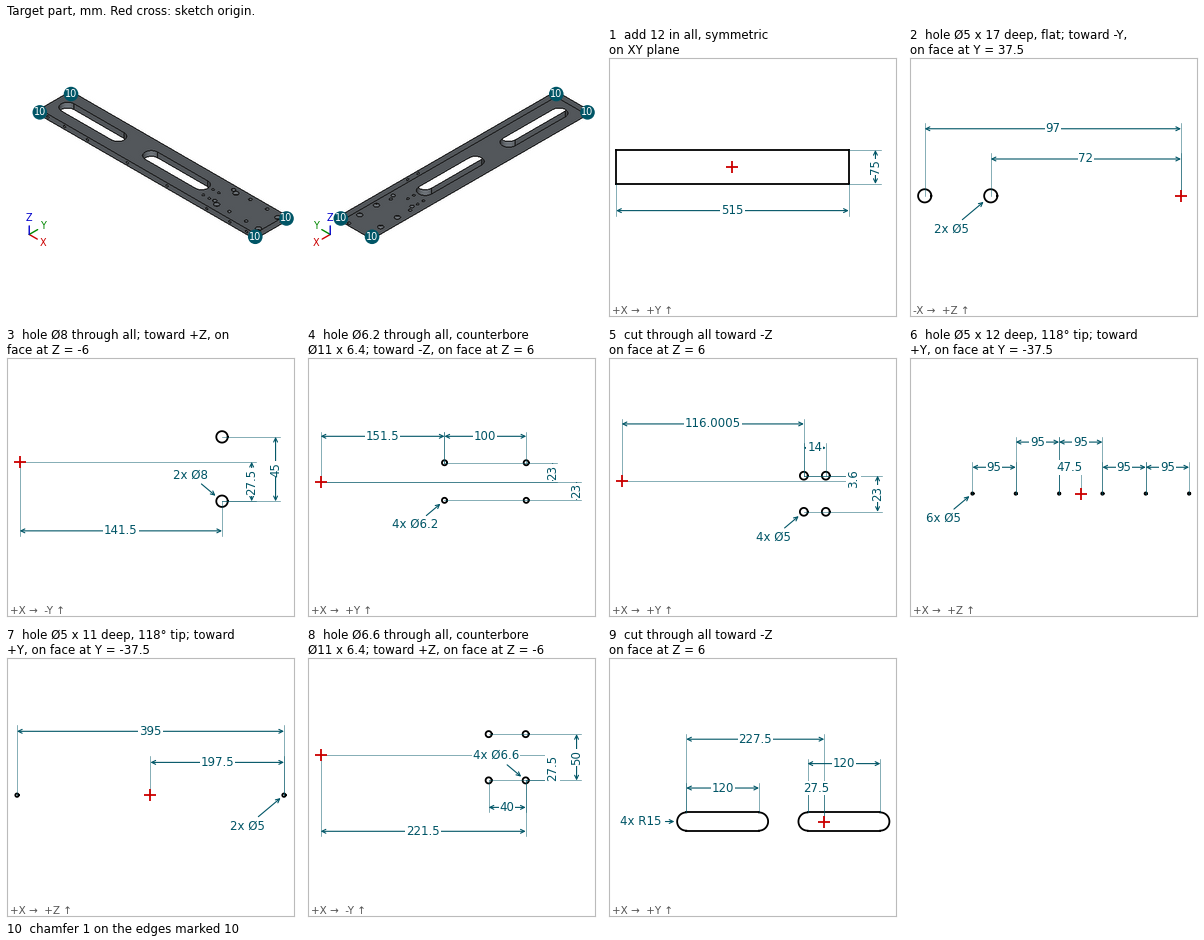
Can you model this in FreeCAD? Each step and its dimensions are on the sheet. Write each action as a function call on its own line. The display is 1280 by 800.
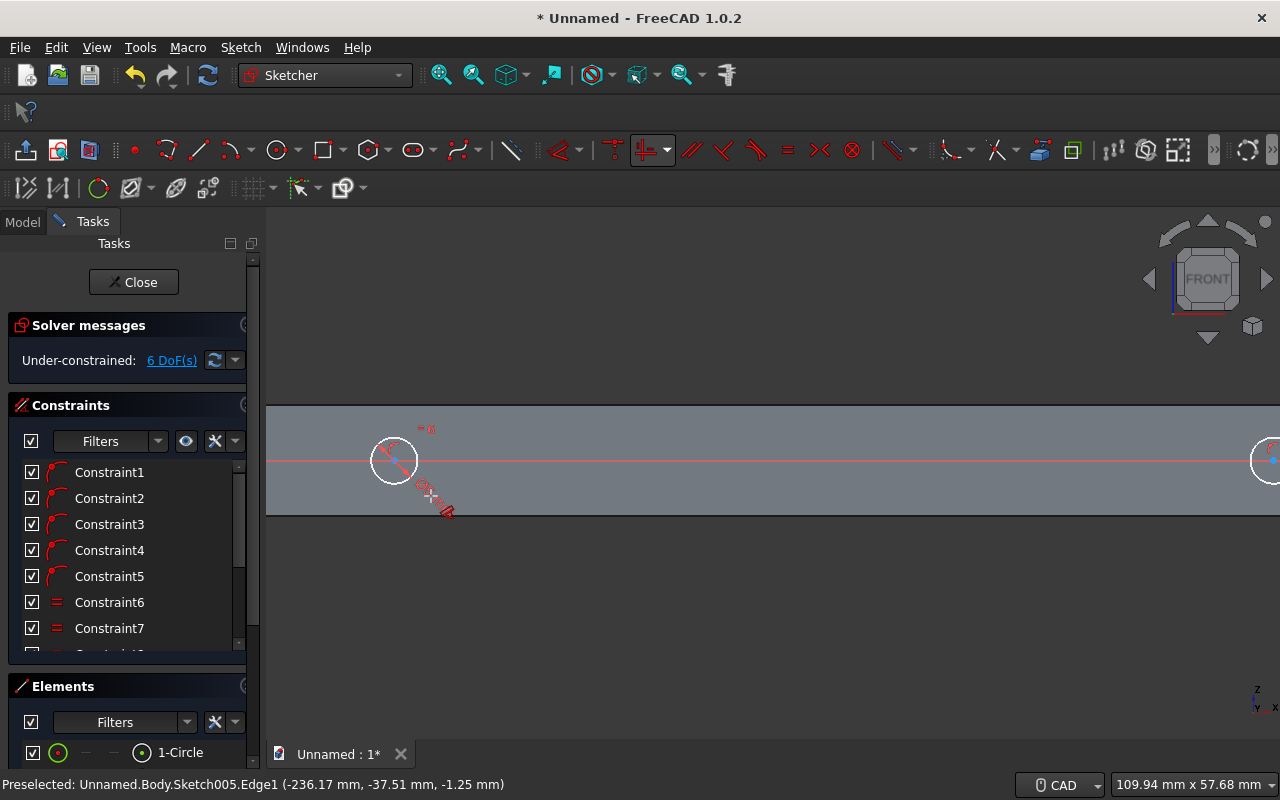
scroll(410, 475, down, 10)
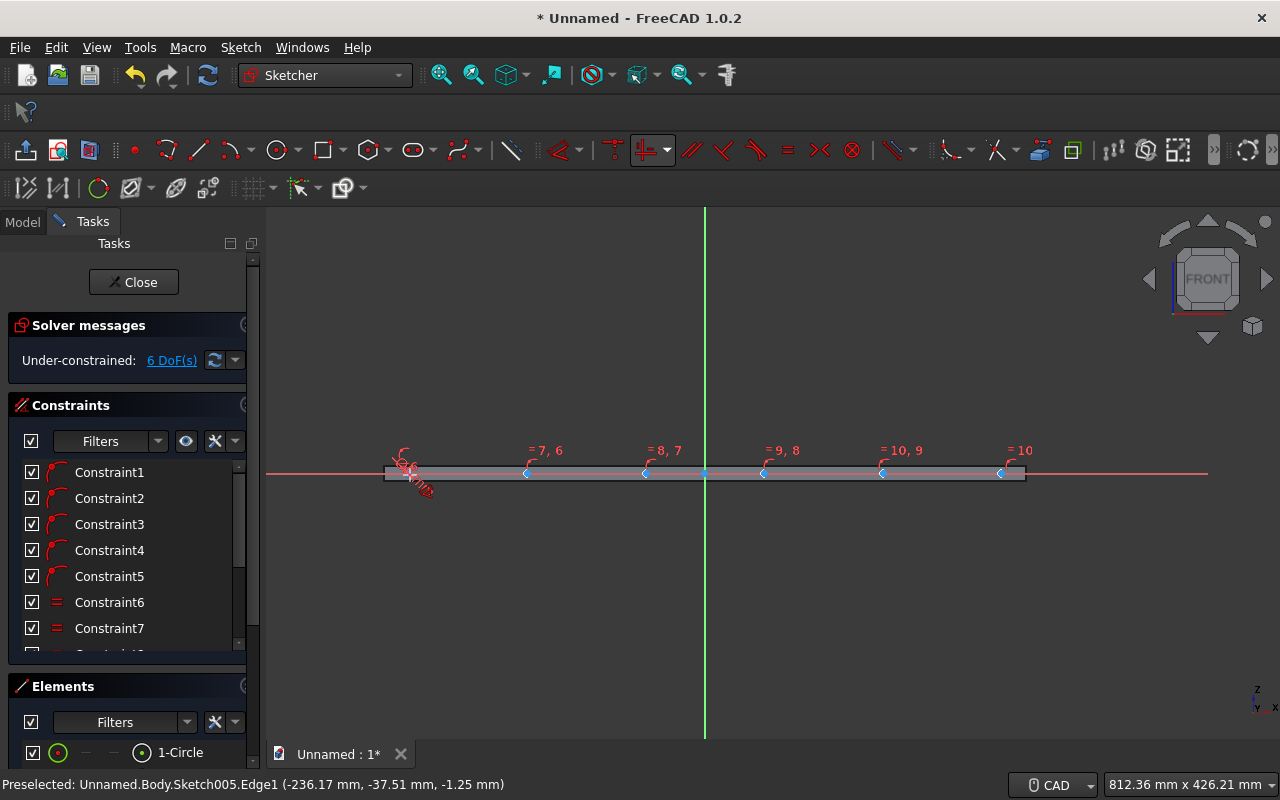
click(408, 473)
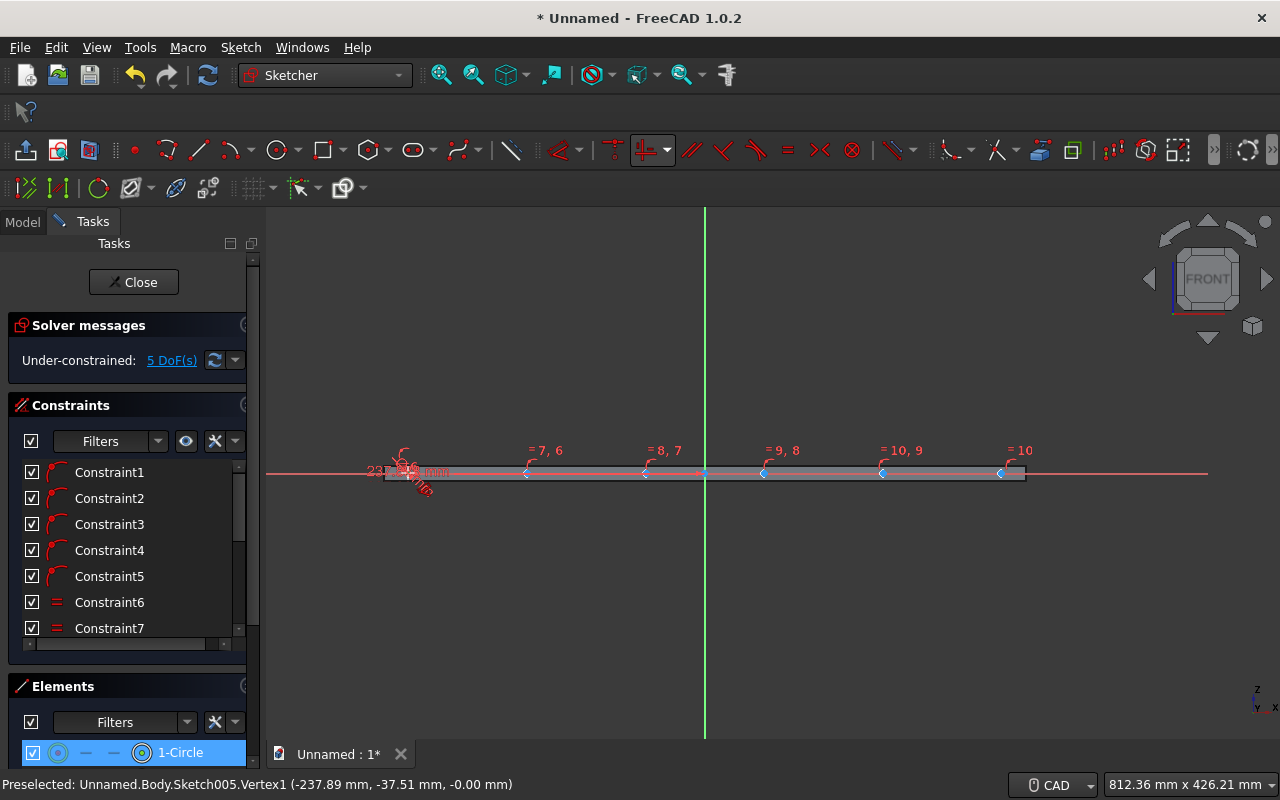
click(527, 473)
click(468, 507)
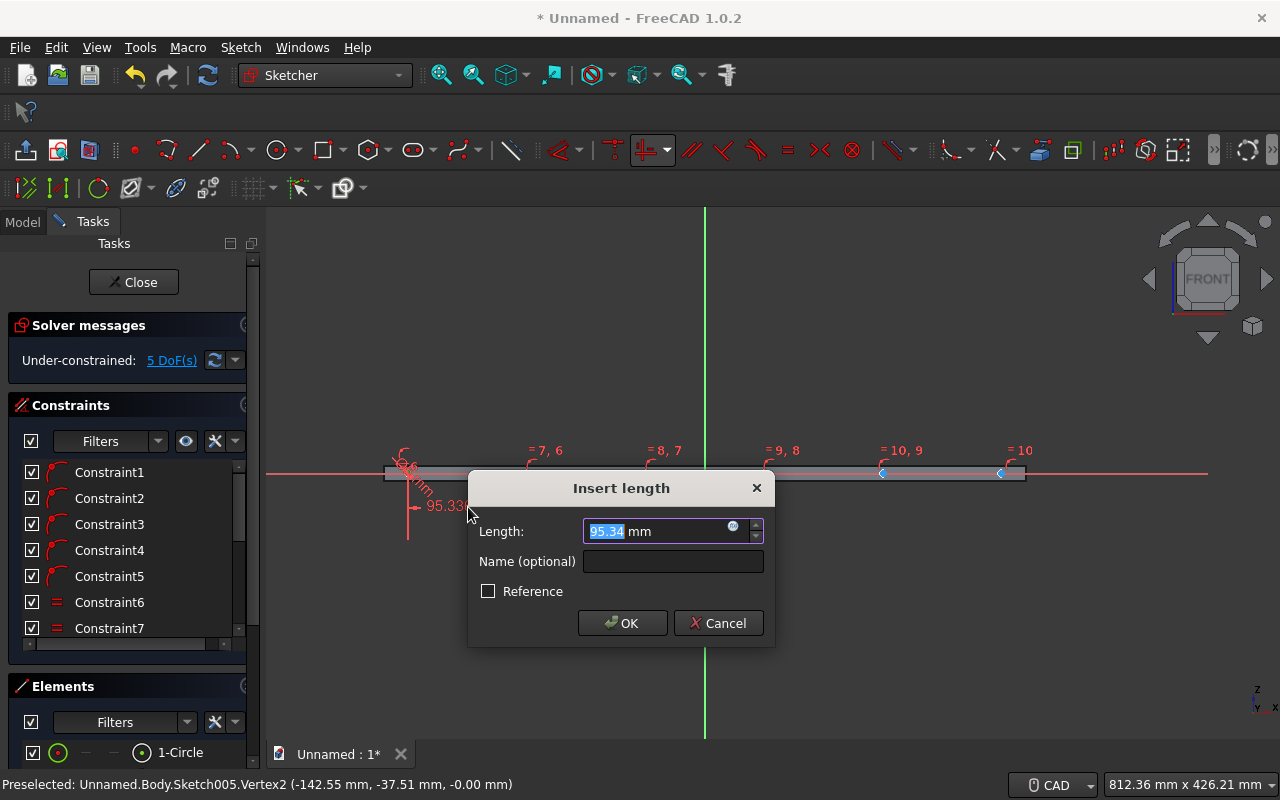
text(95)
key(Return)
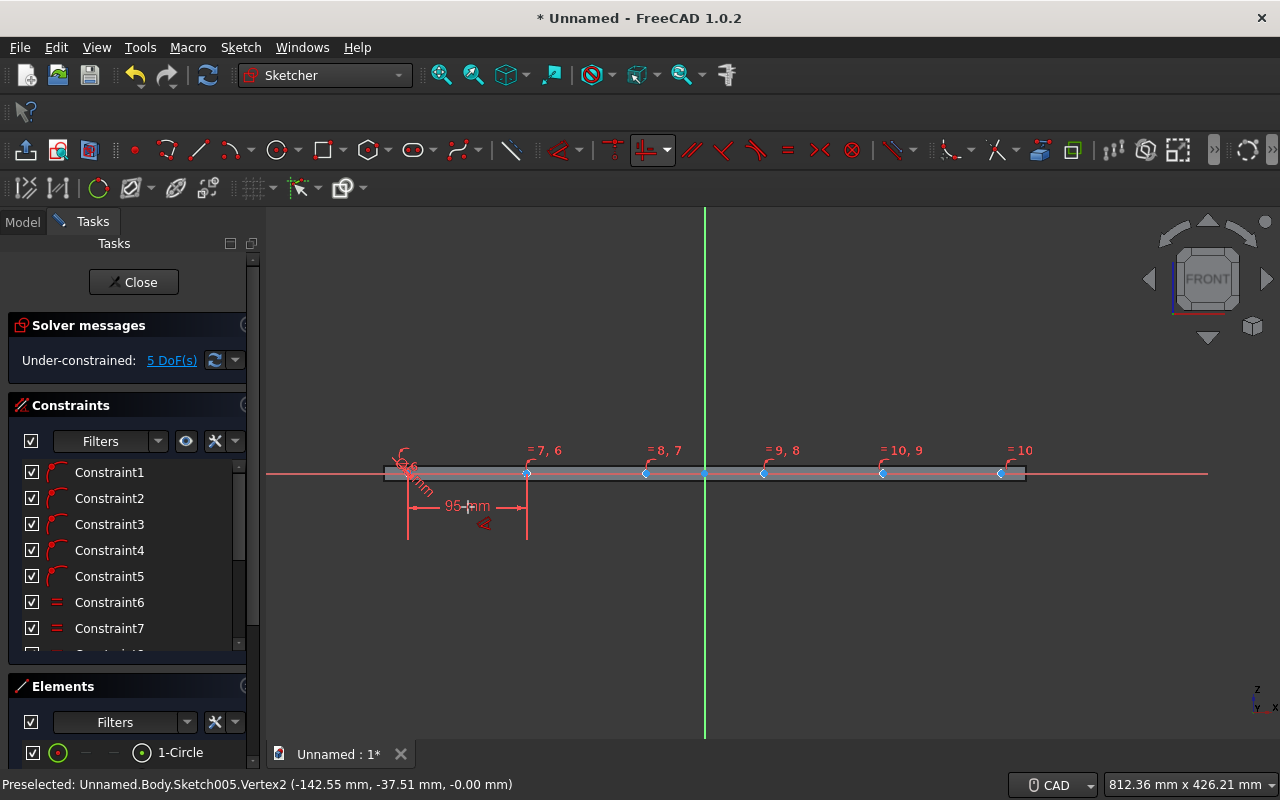
click(527, 473)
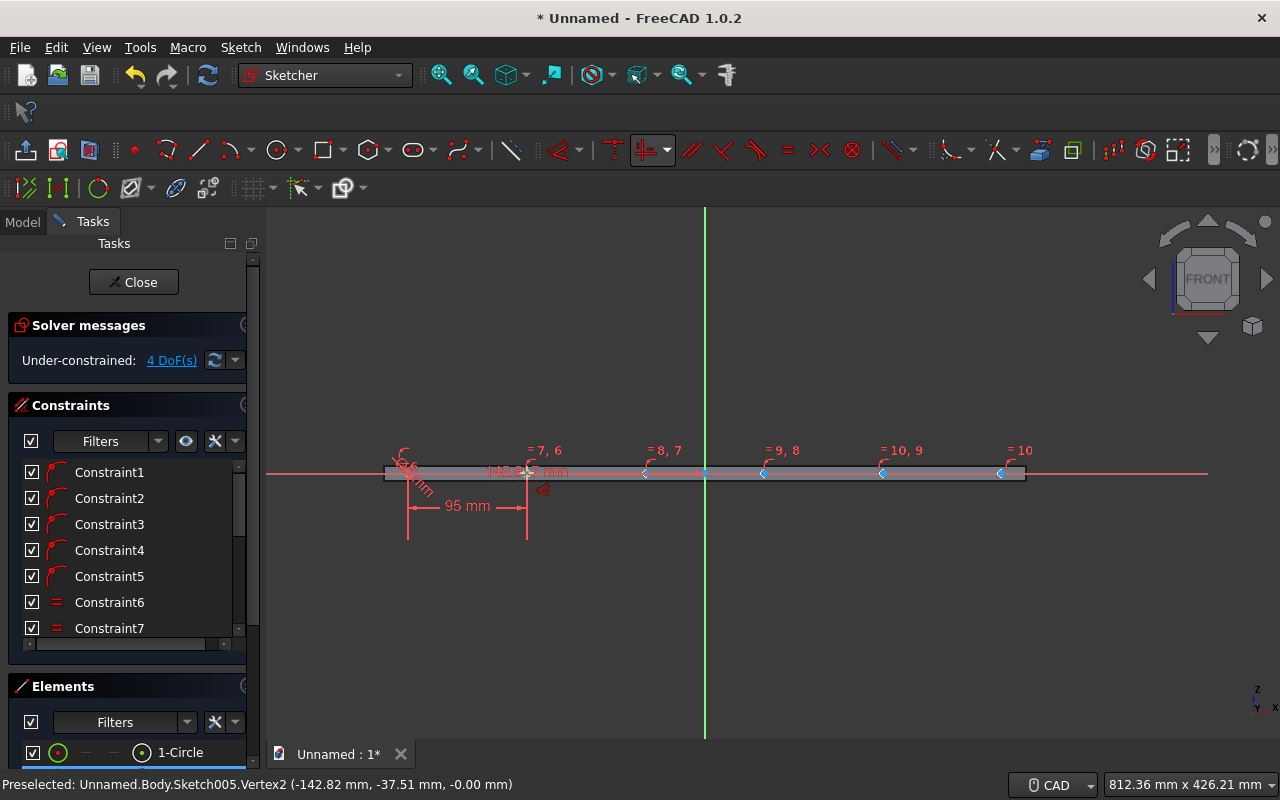
click(646, 473)
click(586, 507)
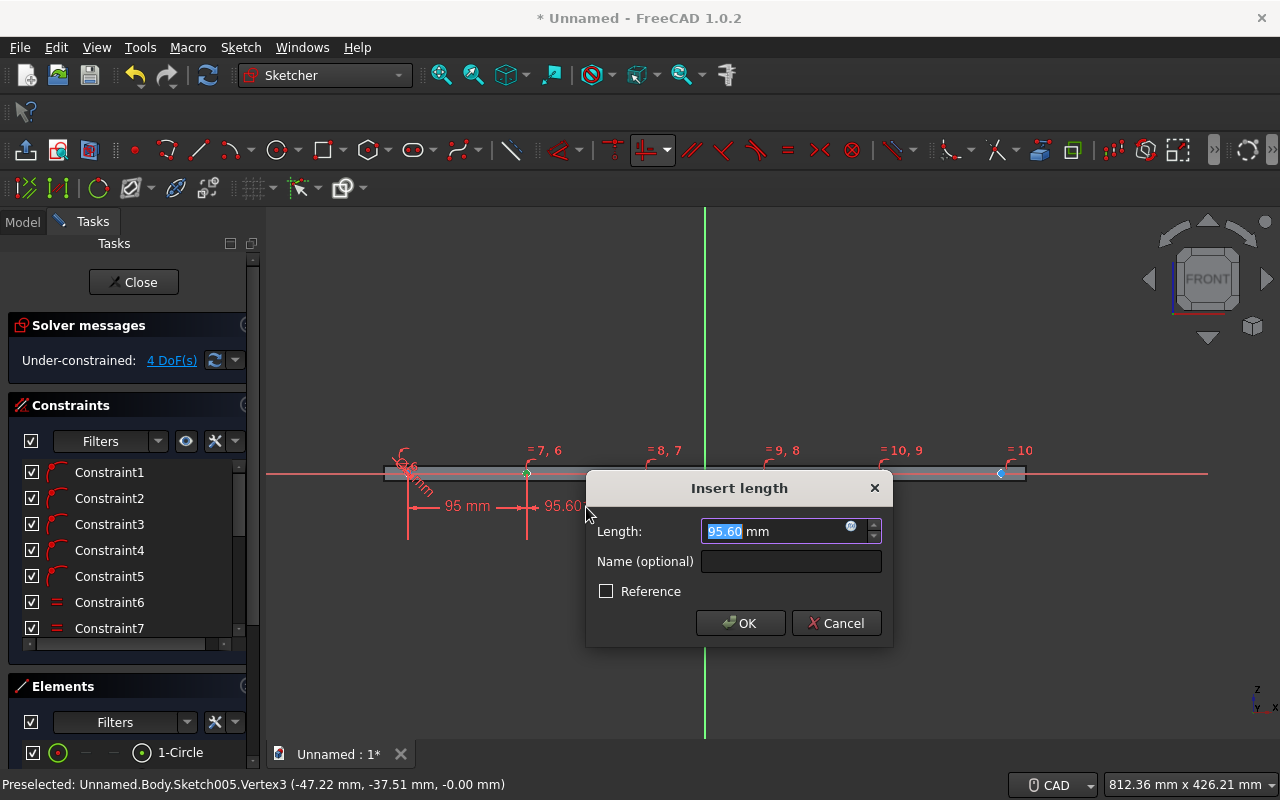
text(95)
key(Return)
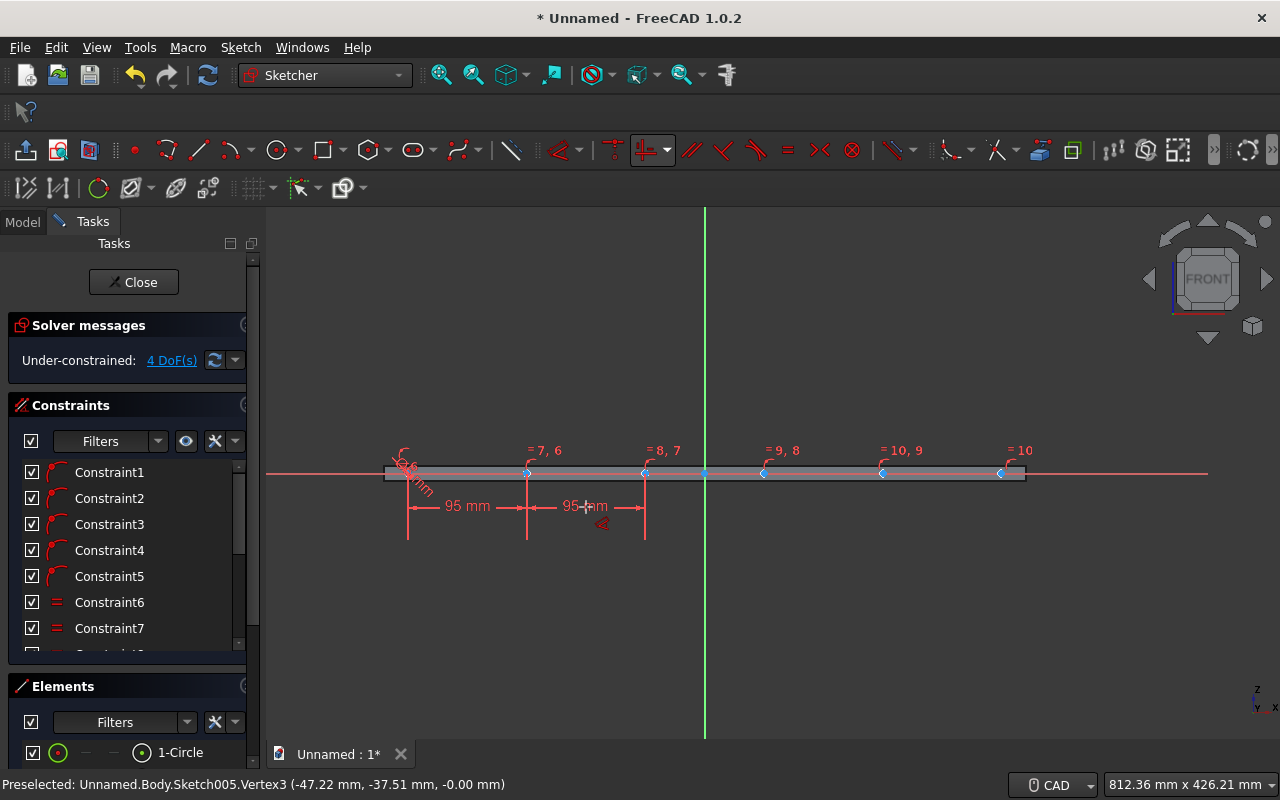
click(645, 473)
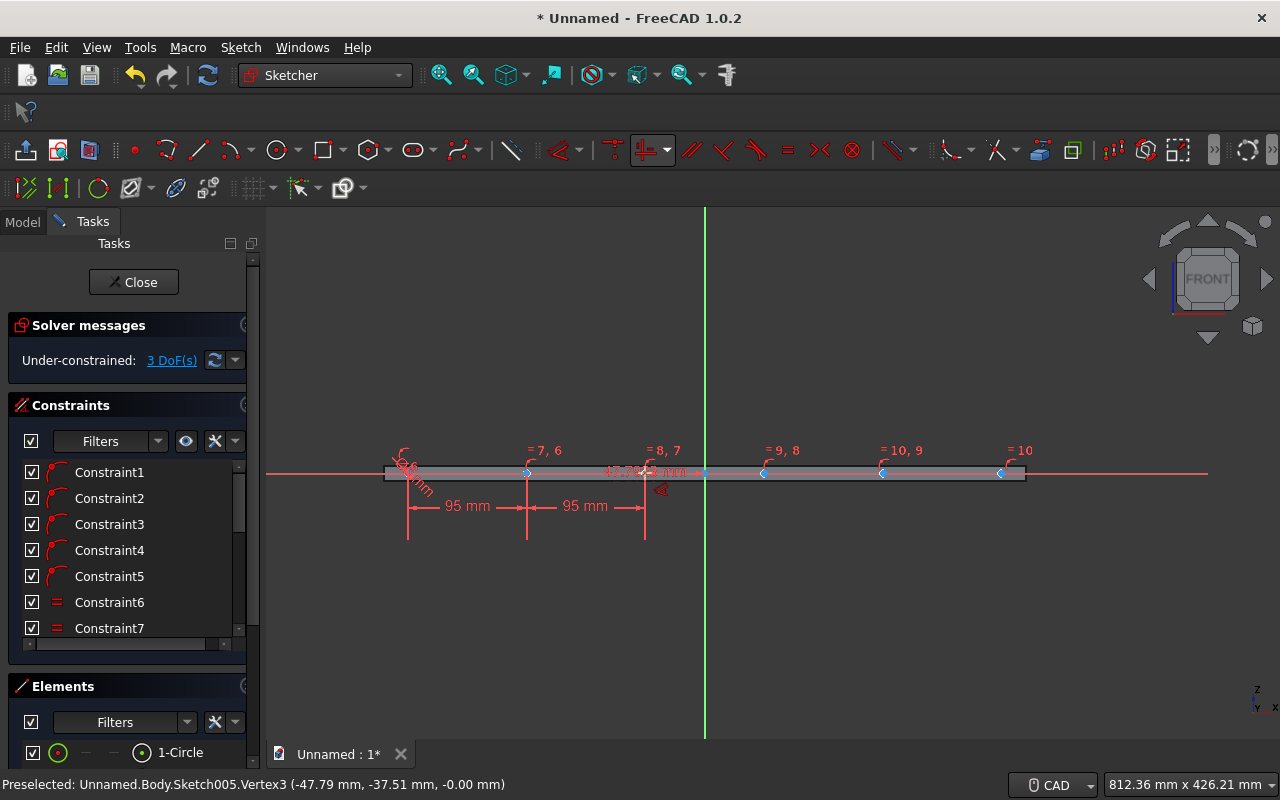
click(764, 473)
click(677, 507)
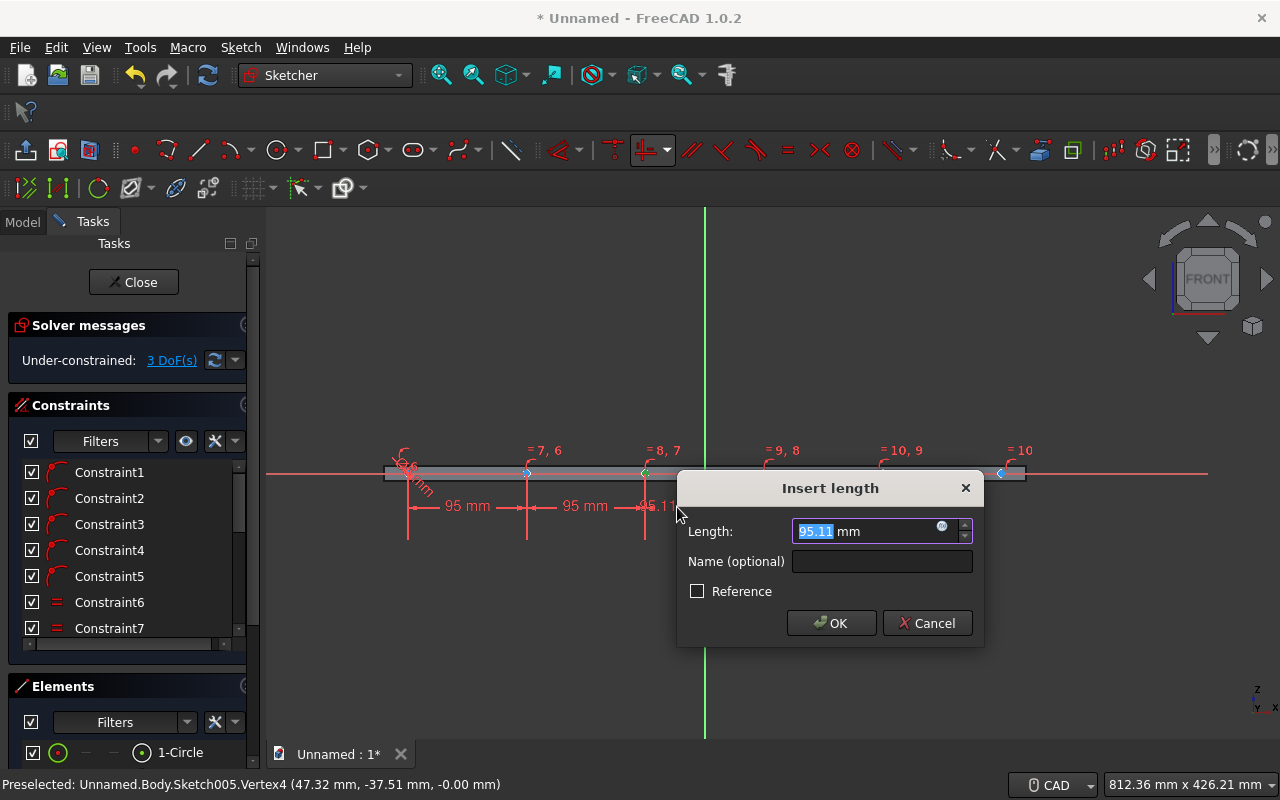
text(95)
key(Return)